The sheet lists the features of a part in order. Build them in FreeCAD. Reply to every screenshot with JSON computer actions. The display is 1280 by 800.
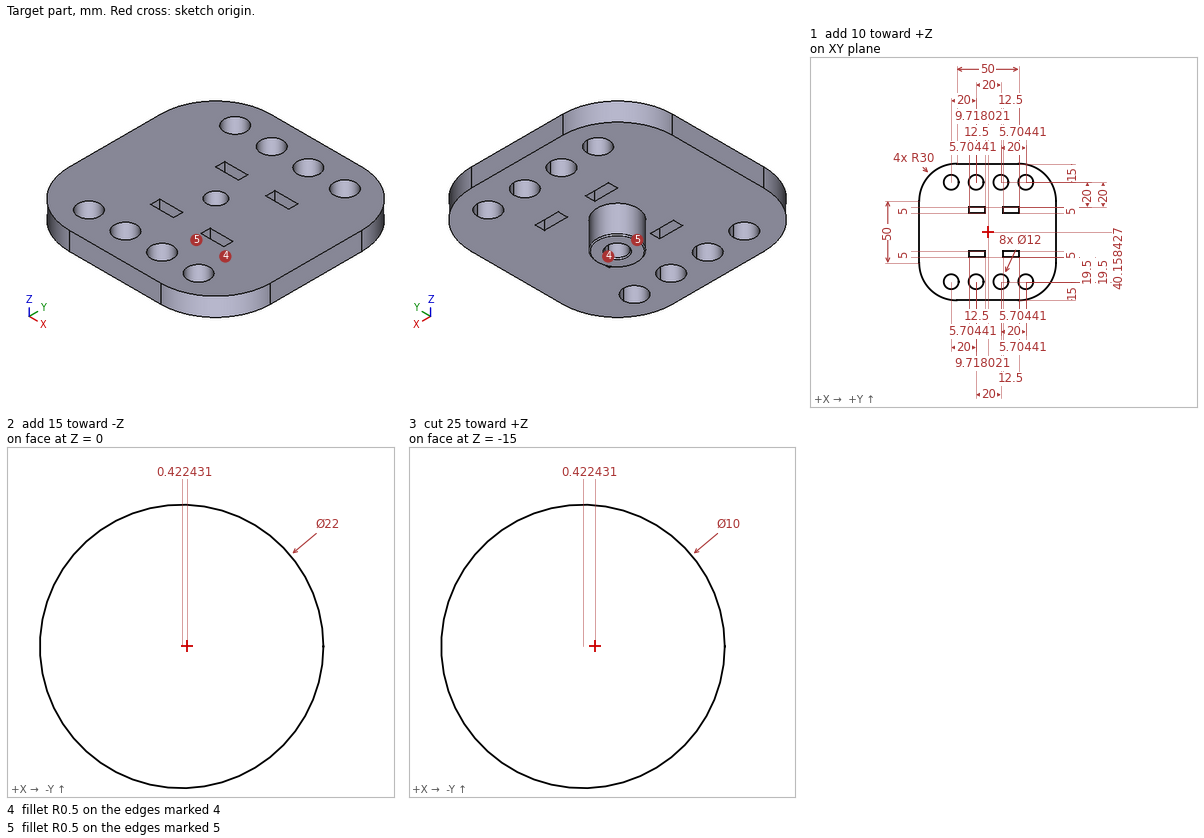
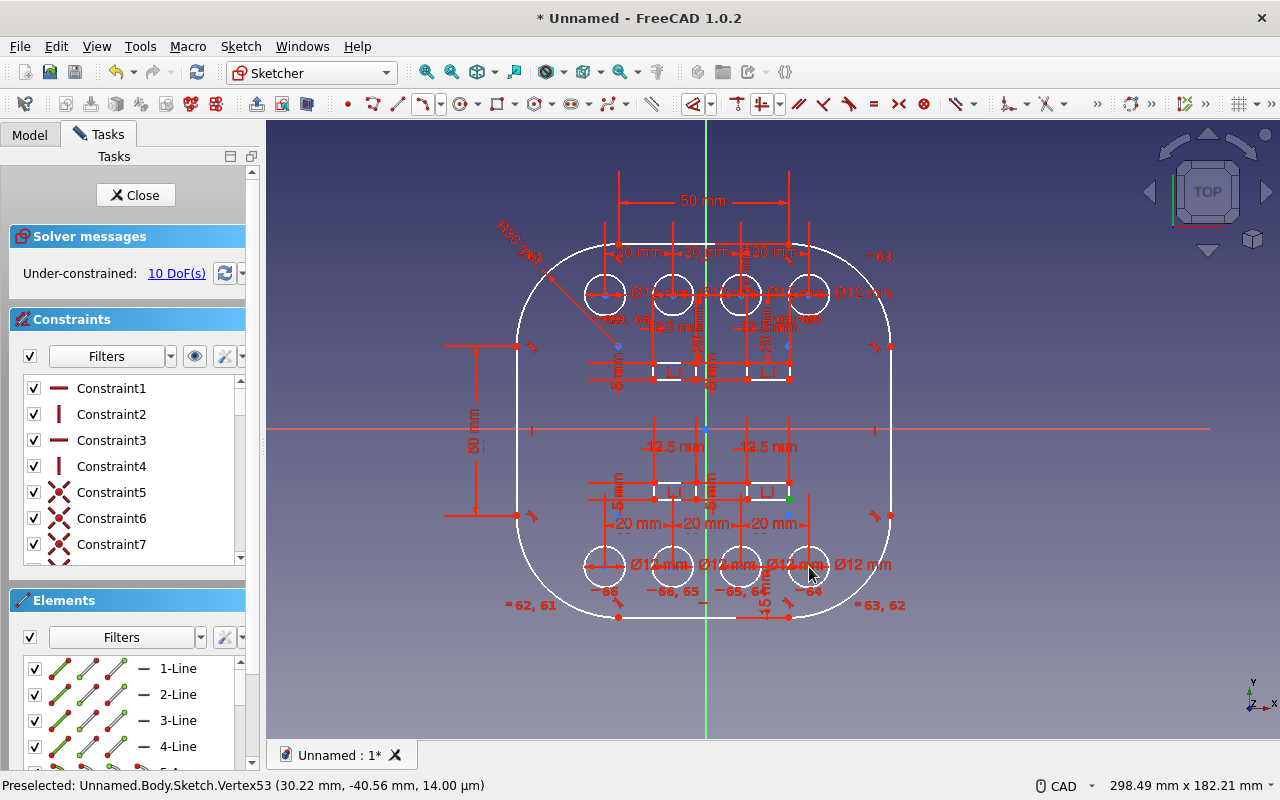
{"action": "key", "text": "i"}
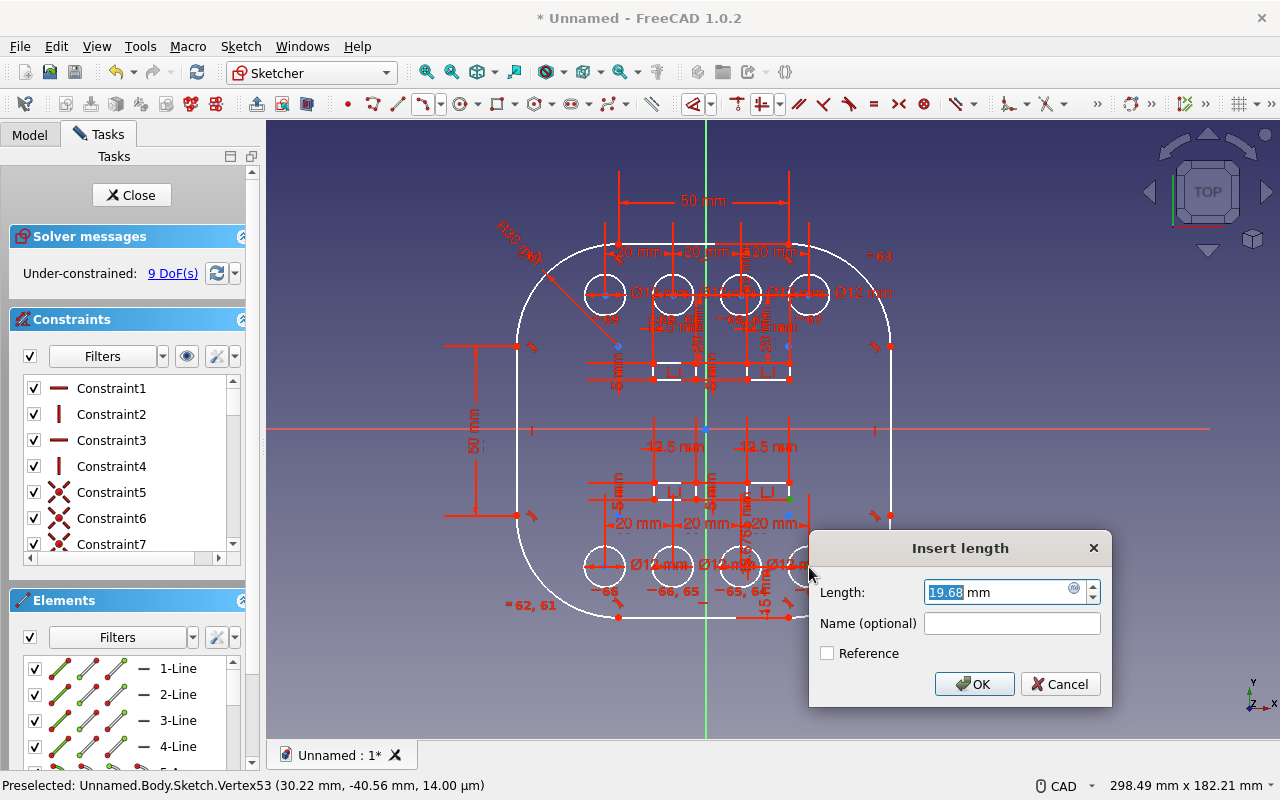
{"action": "type", "text": "19.5"}
{"action": "key", "text": "Return"}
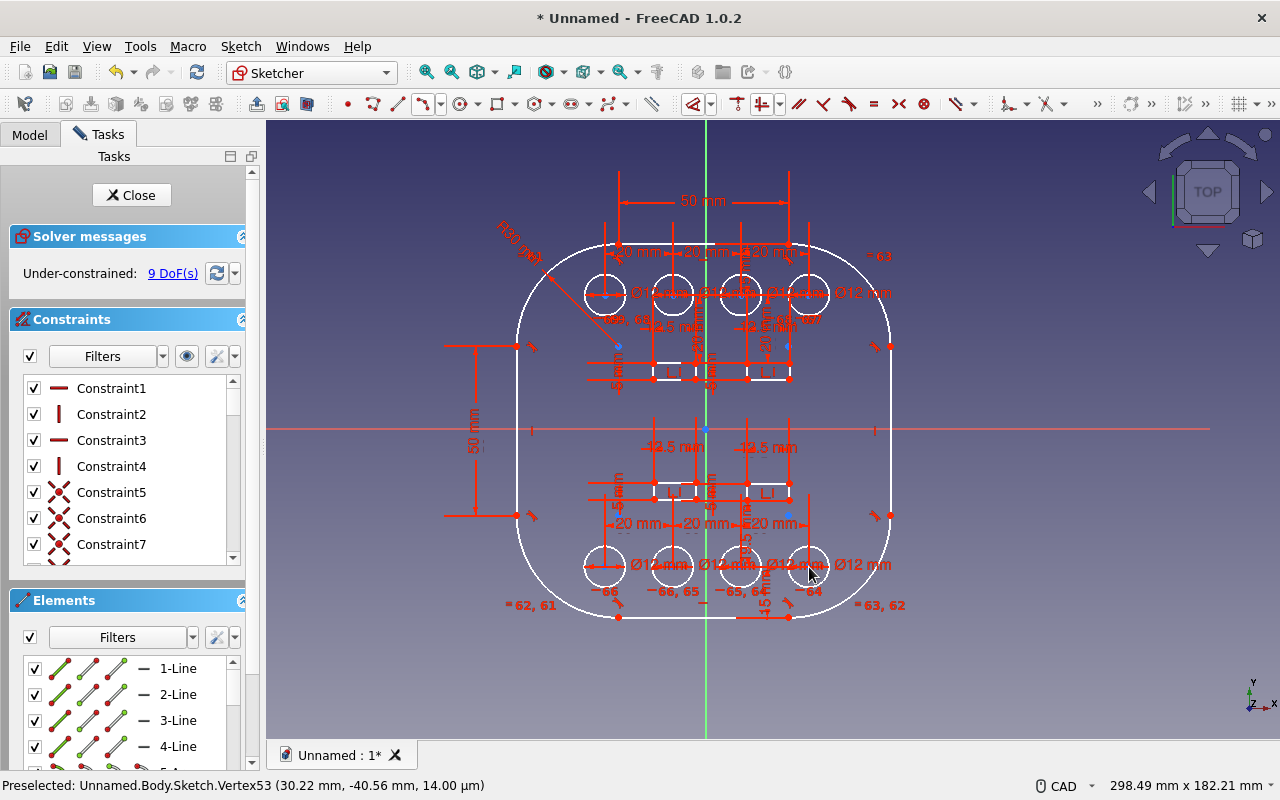
{"action": "left_click", "coordinate": [696, 500]}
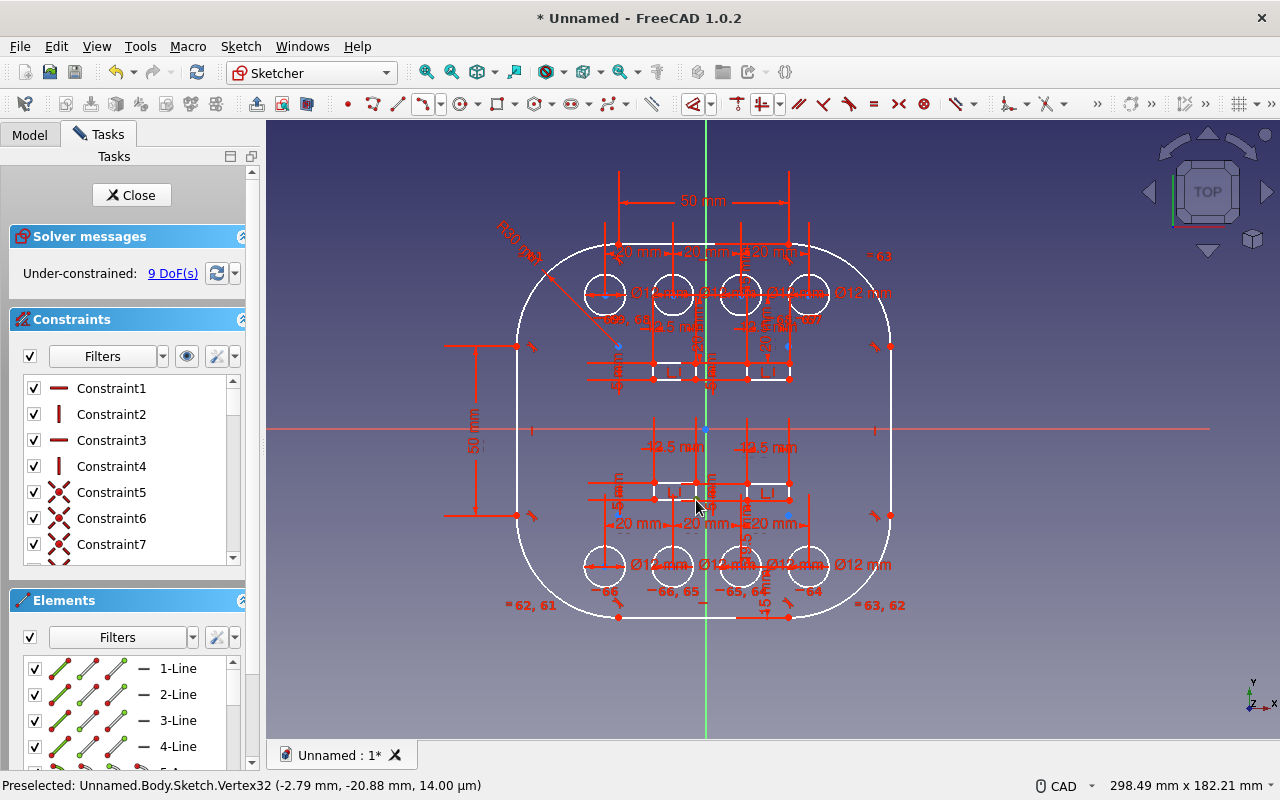
{"action": "left_click", "coordinate": [741, 567]}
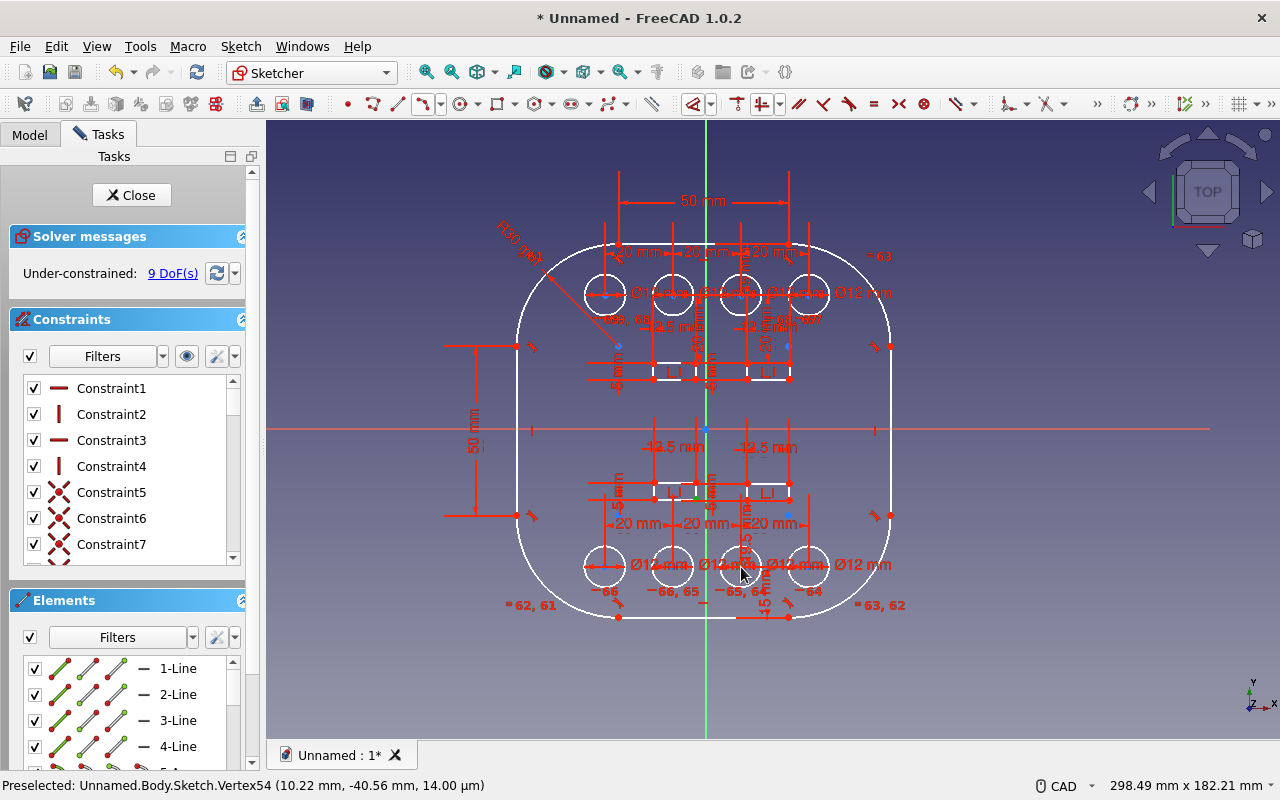
{"action": "left_click", "coordinate": [710, 104]}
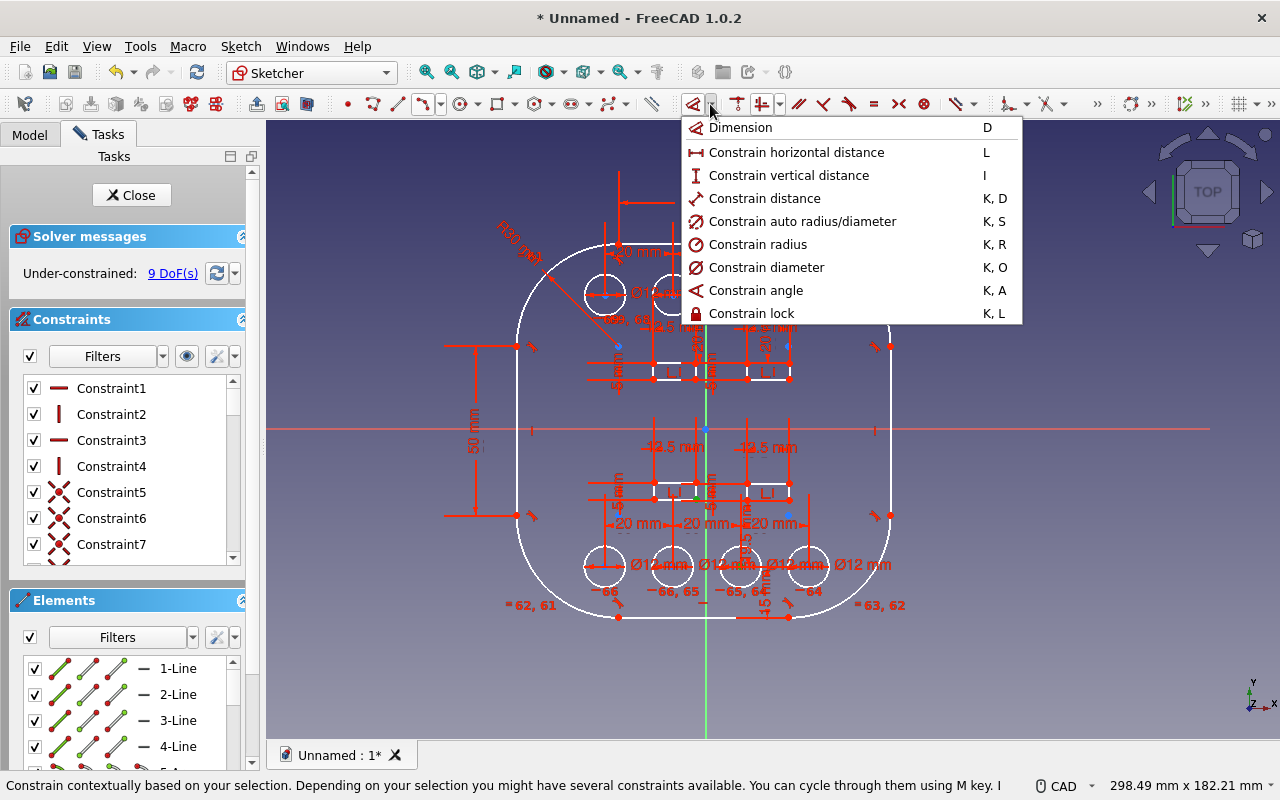
{"action": "left_click", "coordinate": [852, 176]}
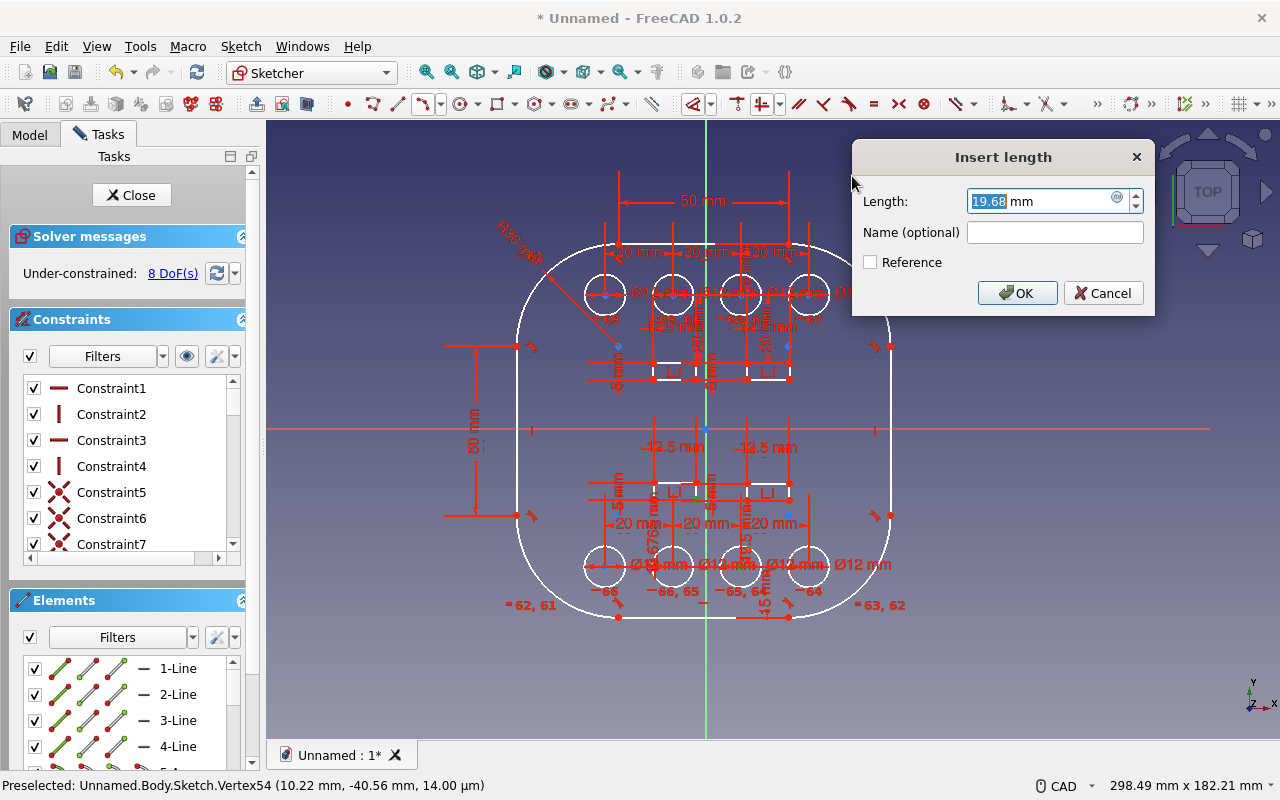
{"action": "type", "text": "19.5"}
{"action": "key", "text": "Return"}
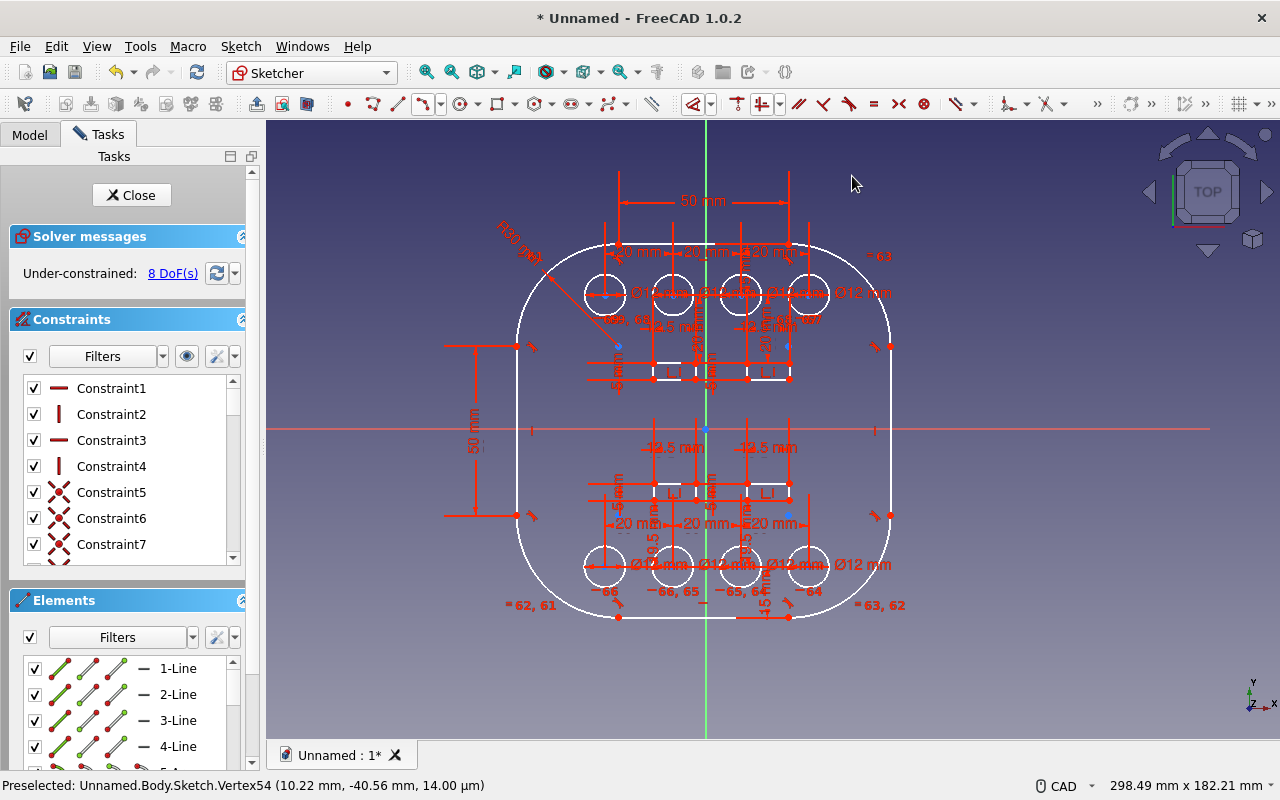
{"action": "left_click", "coordinate": [673, 567]}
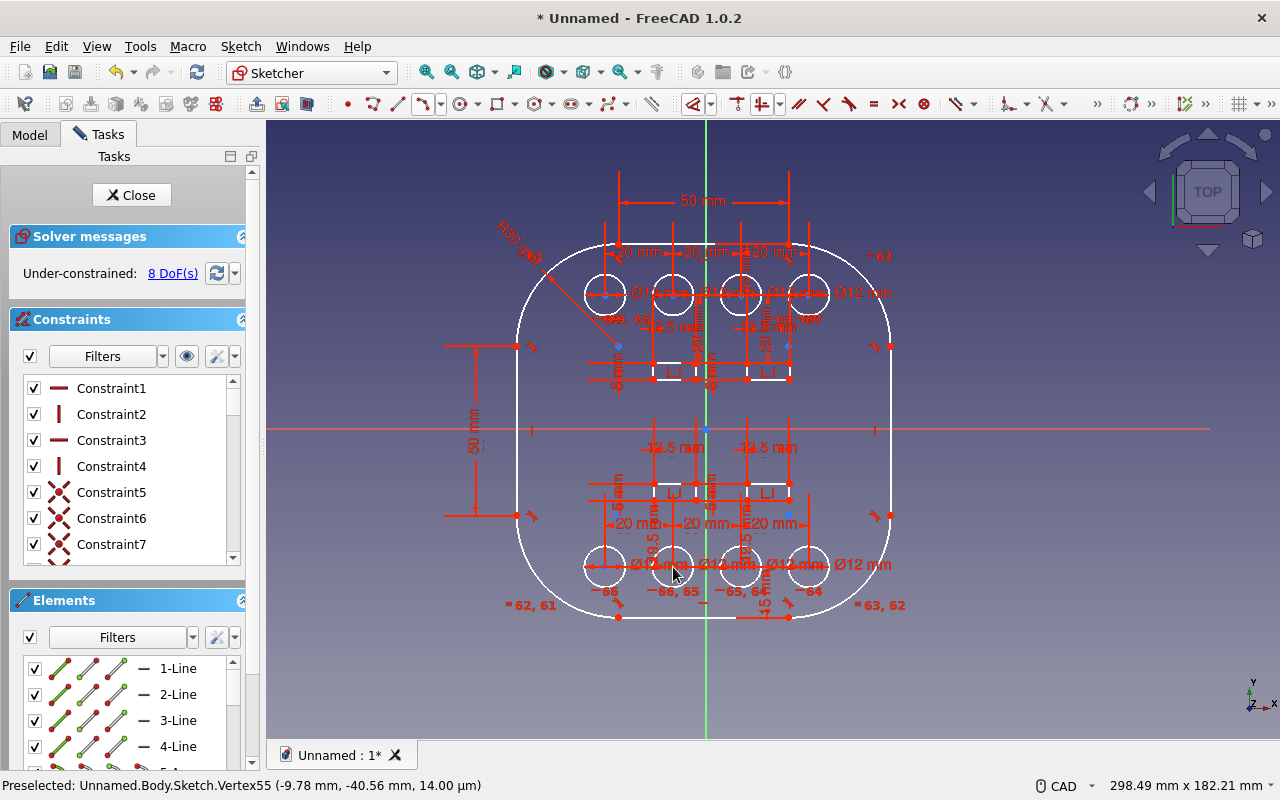
{"action": "key", "text": "l"}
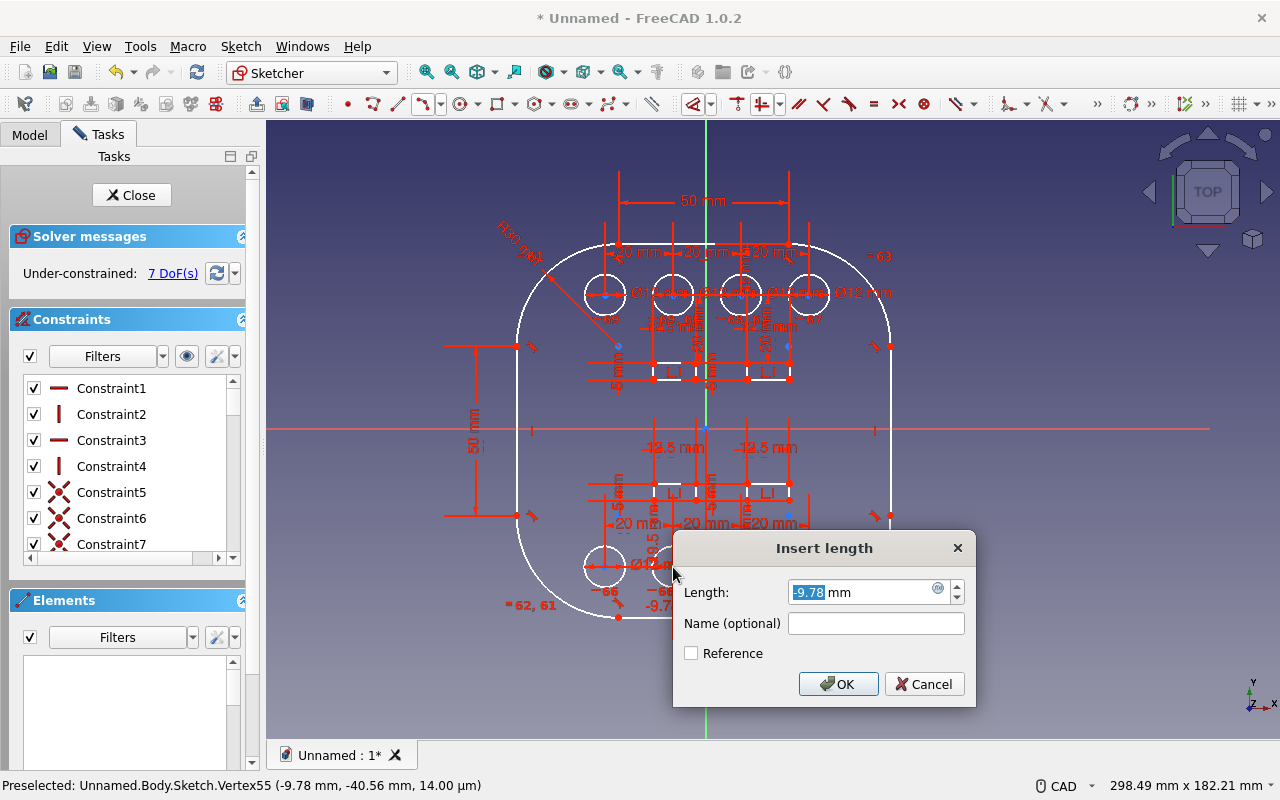
{"action": "type", "text": "-9.718021"}
{"action": "key", "text": "Return"}